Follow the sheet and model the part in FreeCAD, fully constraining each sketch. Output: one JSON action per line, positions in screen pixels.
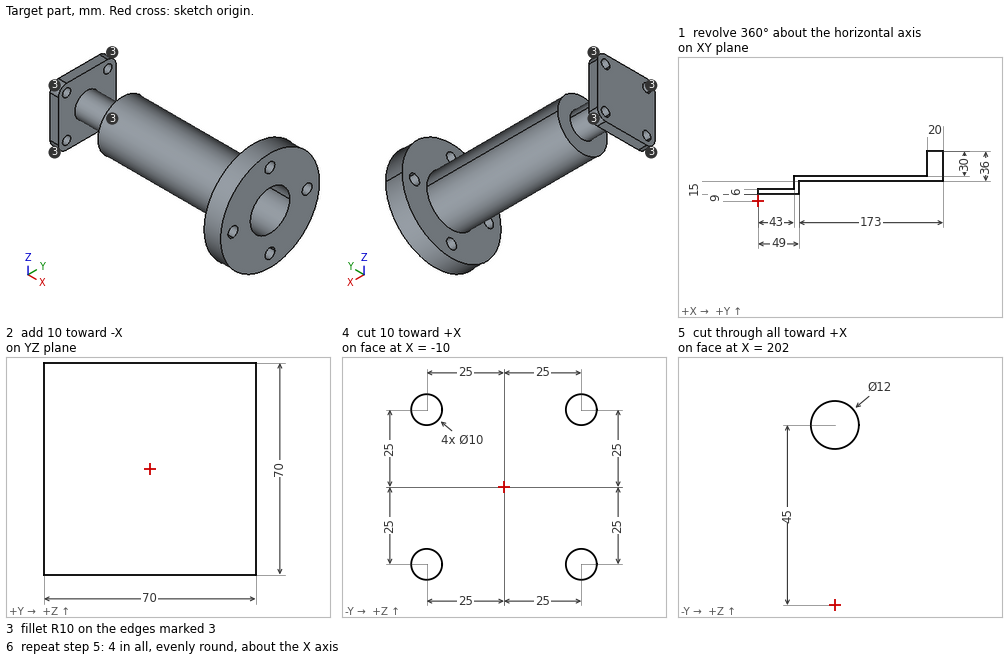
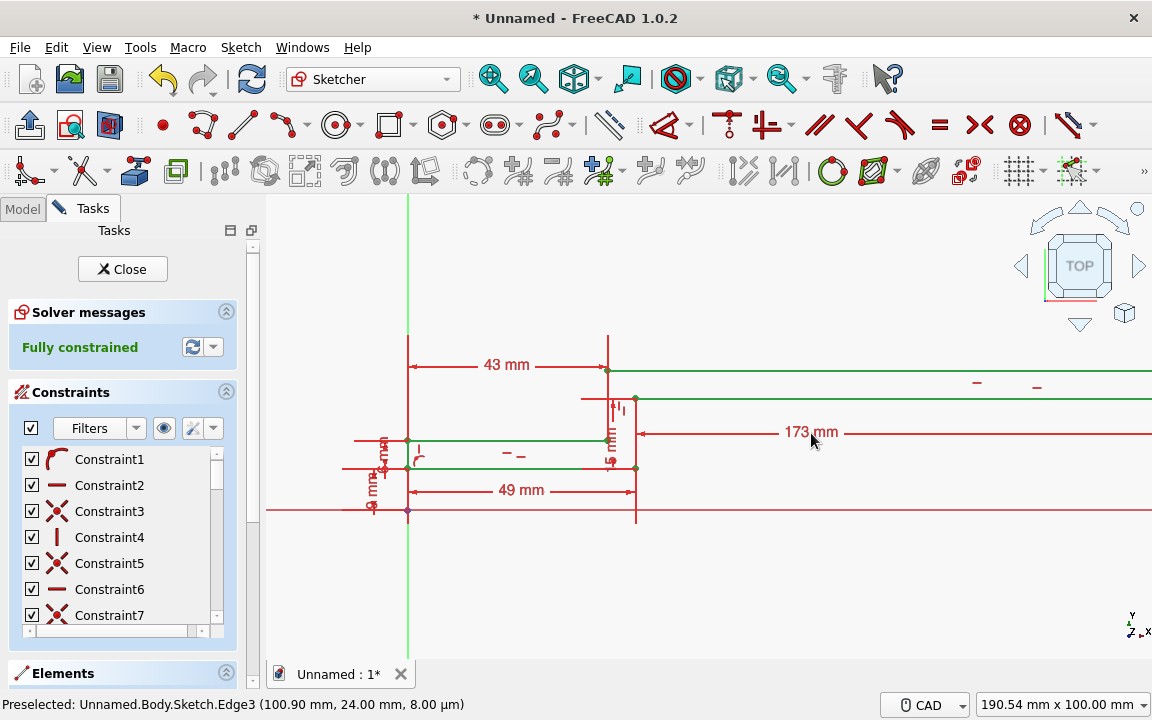
{"action": "left_click", "coordinate": [123, 269]}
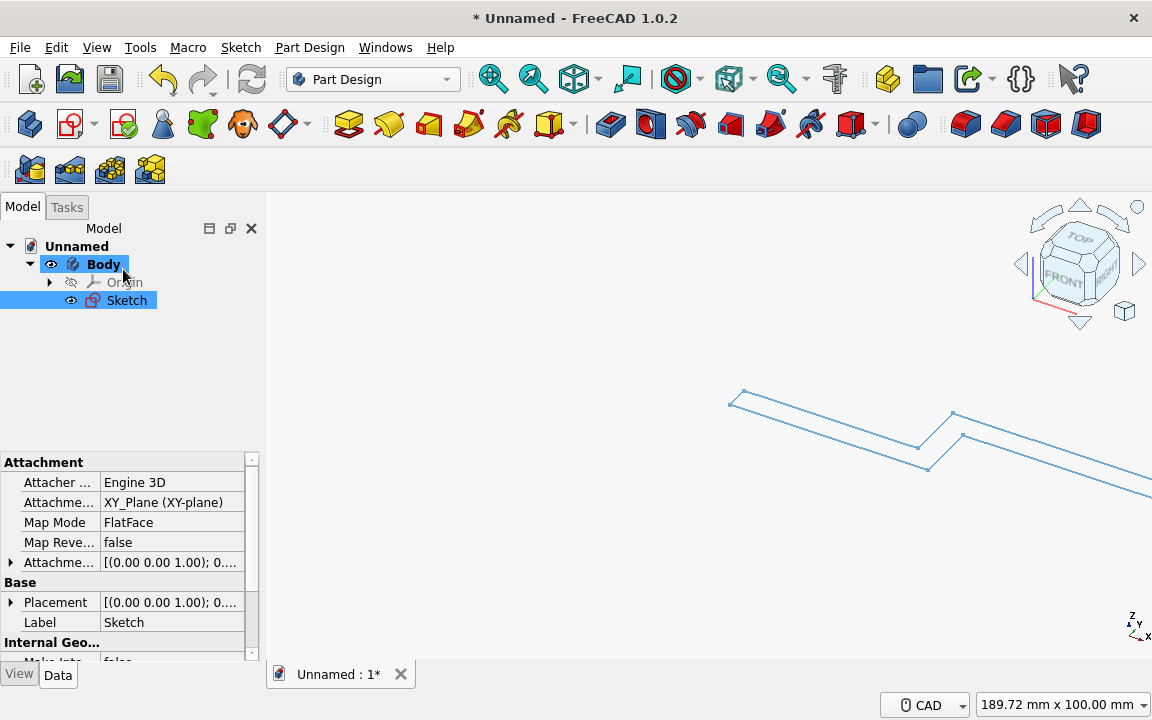
{"action": "left_click", "coordinate": [390, 124]}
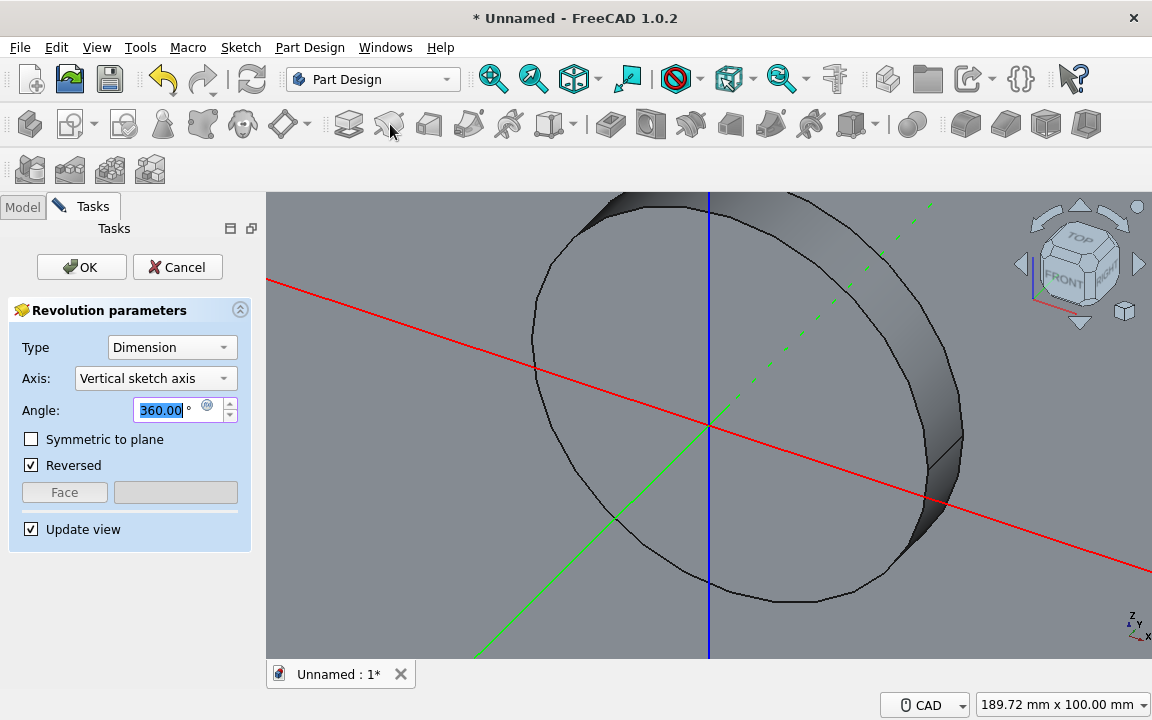
{"action": "left_click", "coordinate": [156, 378]}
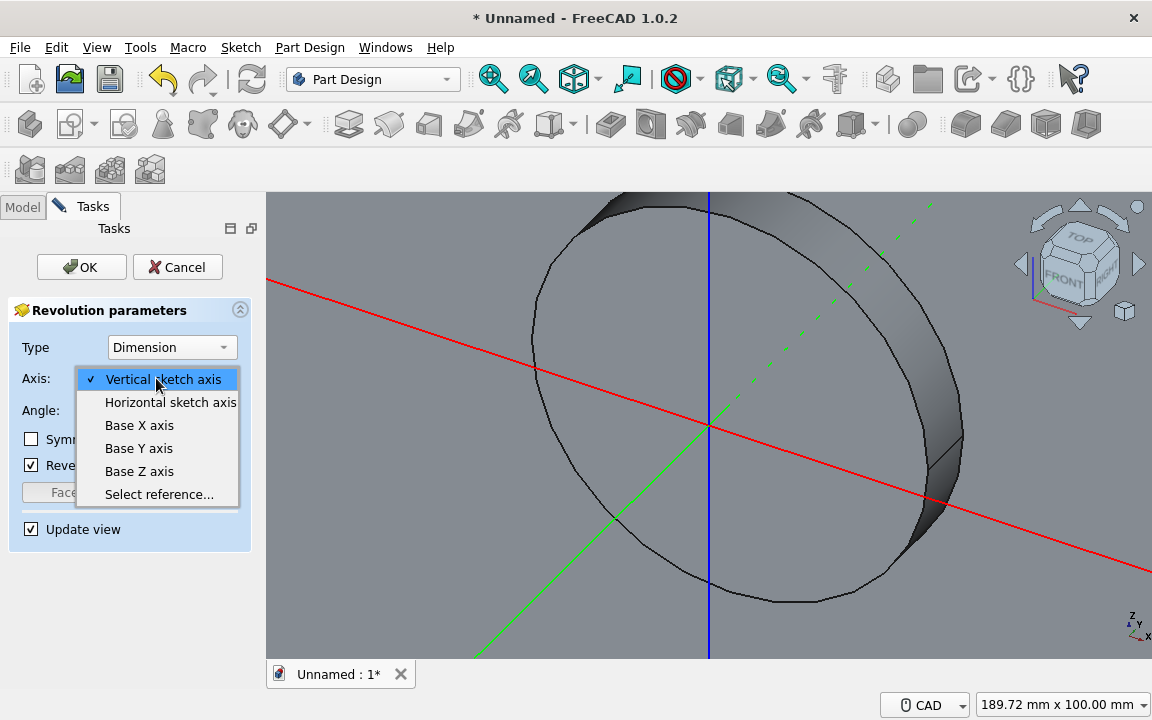
{"action": "left_click", "coordinate": [156, 402]}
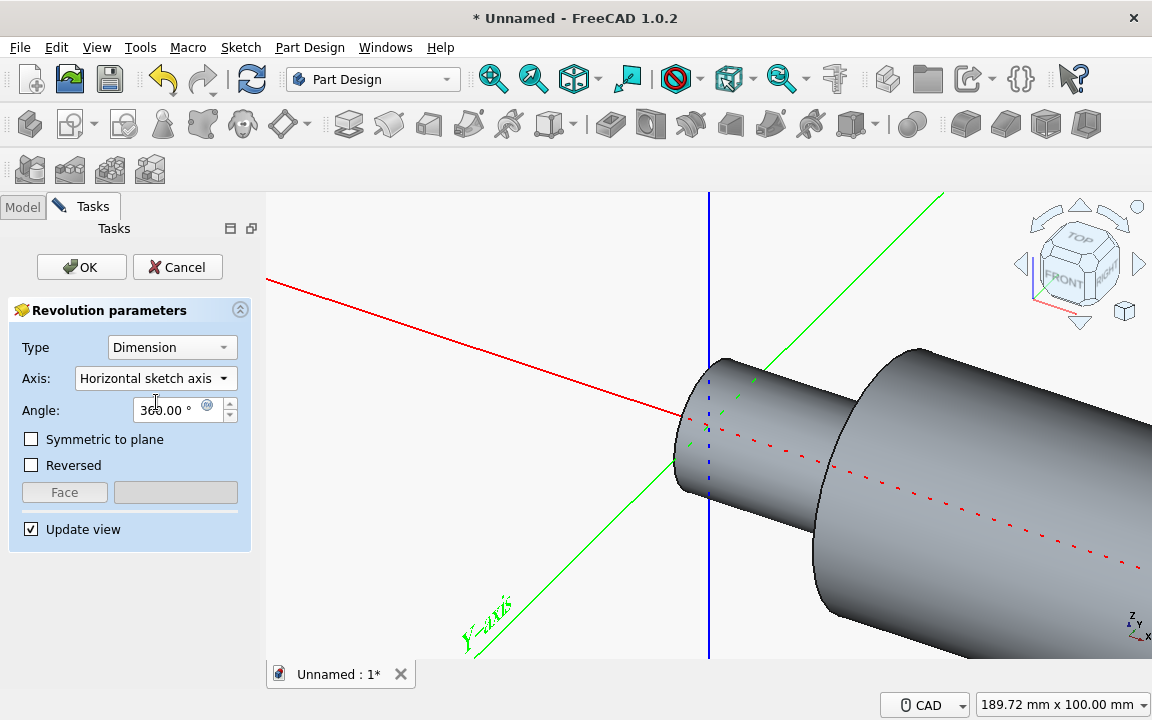
{"action": "left_click", "coordinate": [82, 267]}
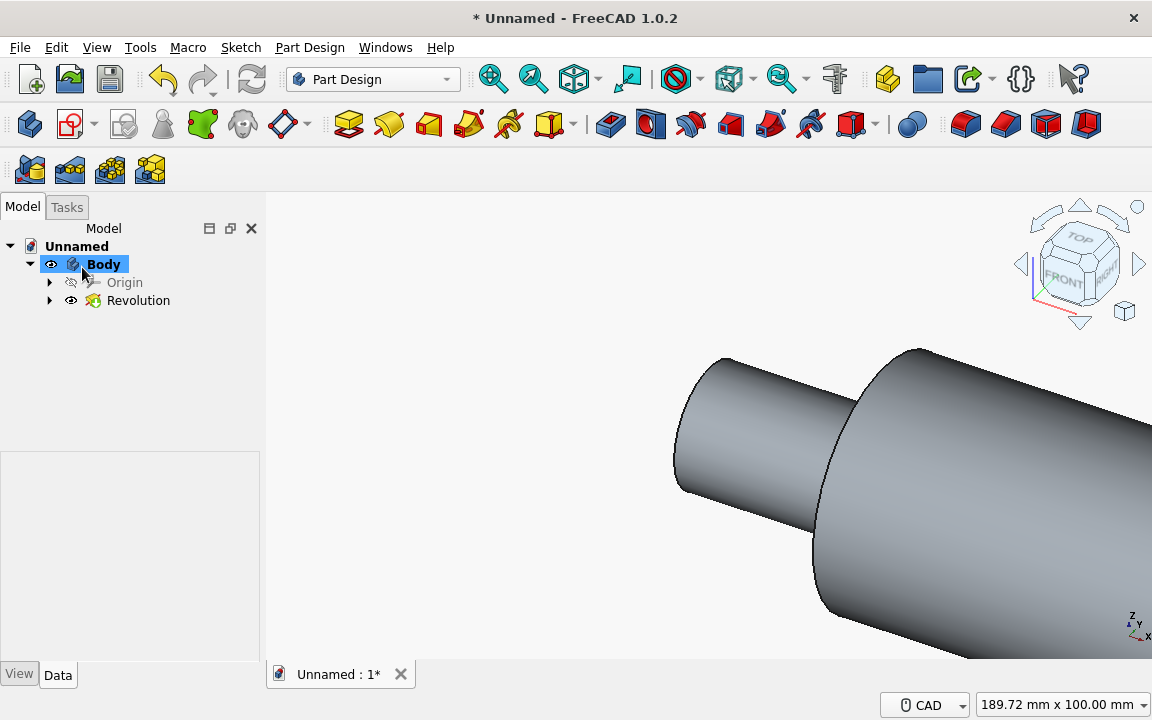
{"action": "left_click", "coordinate": [494, 80]}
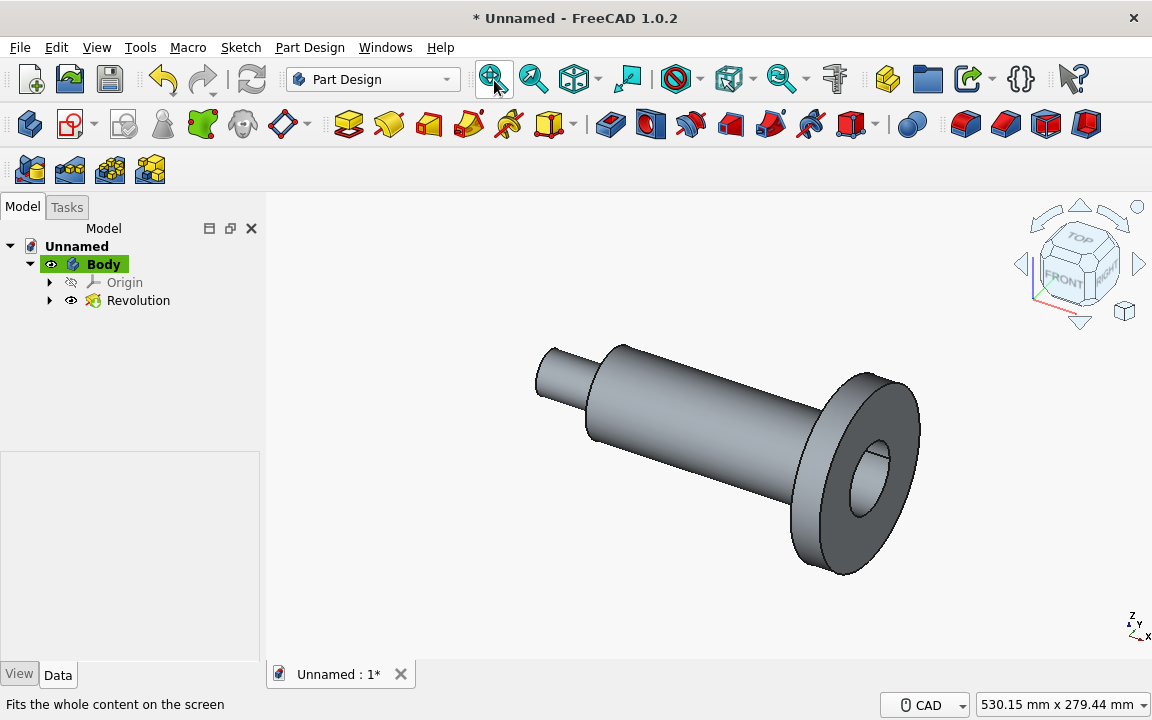
{"action": "left_click", "coordinate": [70, 124]}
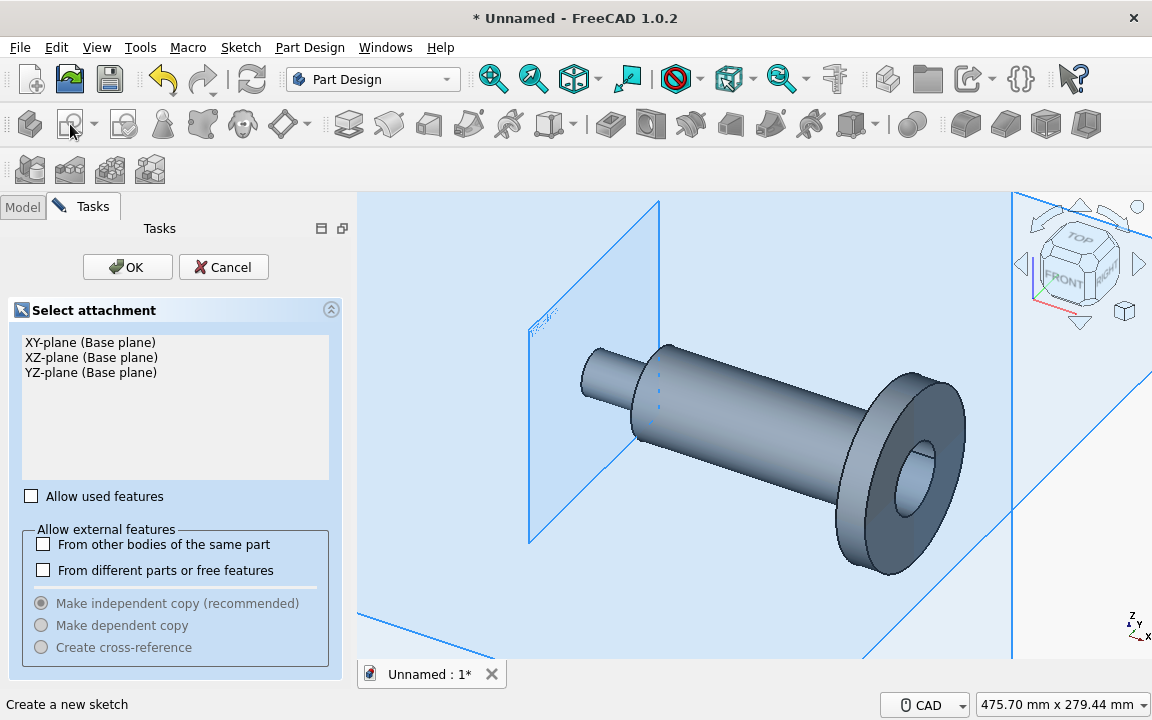
{"action": "left_click", "coordinate": [82, 372]}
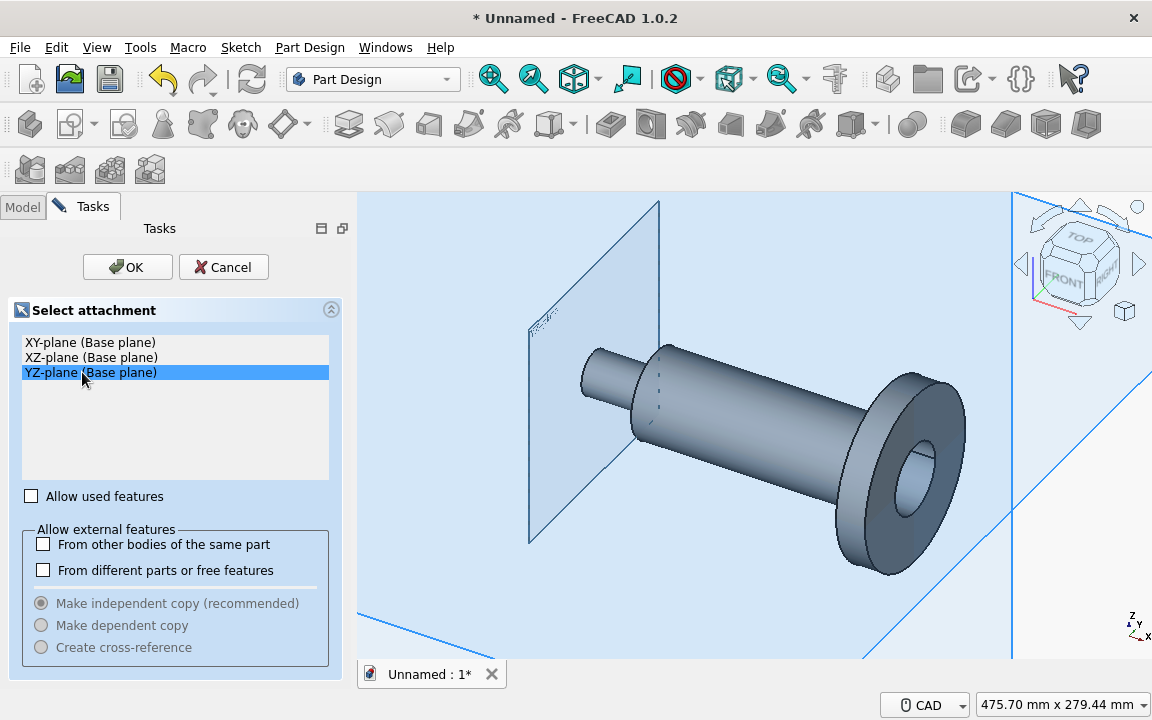
{"action": "left_click", "coordinate": [128, 267]}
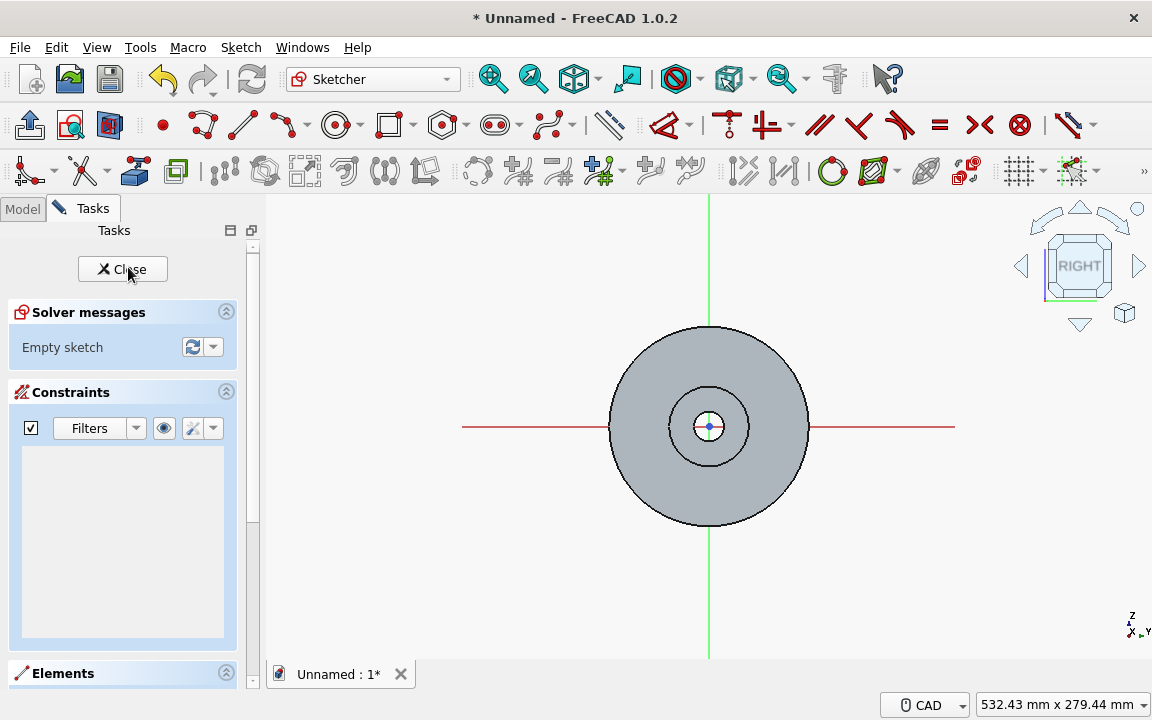
{"action": "left_click", "coordinate": [110, 126]}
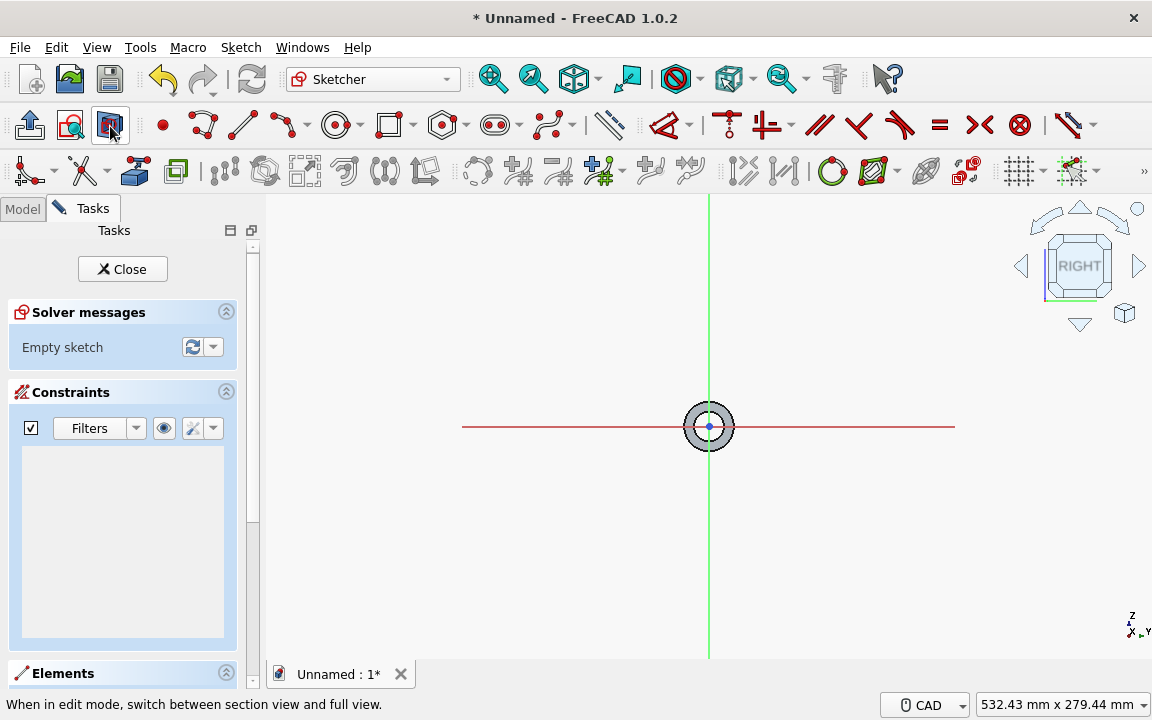
{"action": "scroll", "coordinate": [749, 426], "scroll_direction": "up", "scroll_amount": 5}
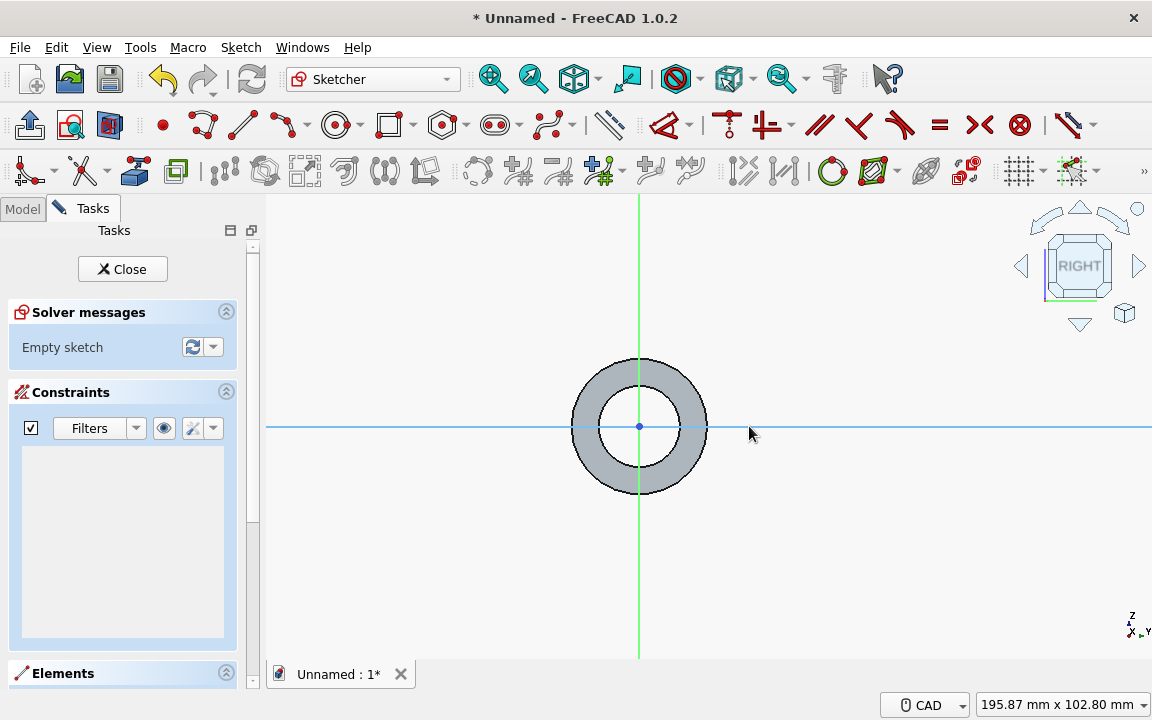
{"action": "key", "text": "g v"}